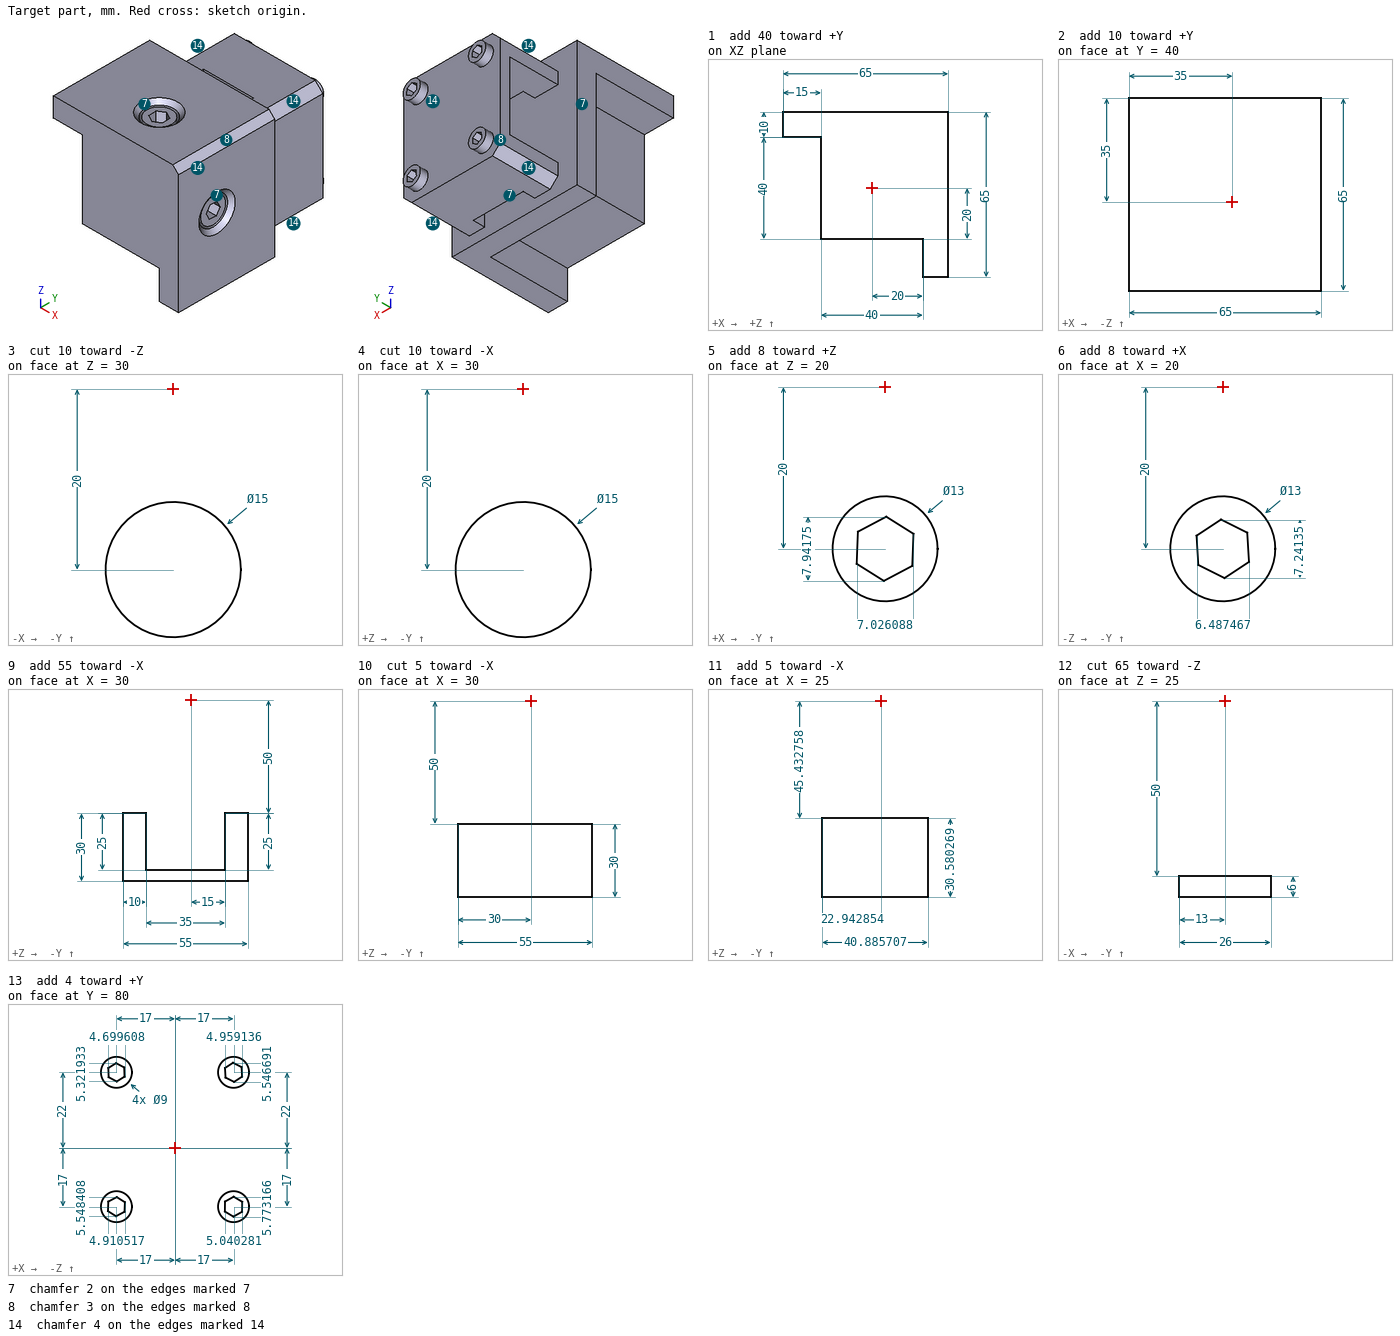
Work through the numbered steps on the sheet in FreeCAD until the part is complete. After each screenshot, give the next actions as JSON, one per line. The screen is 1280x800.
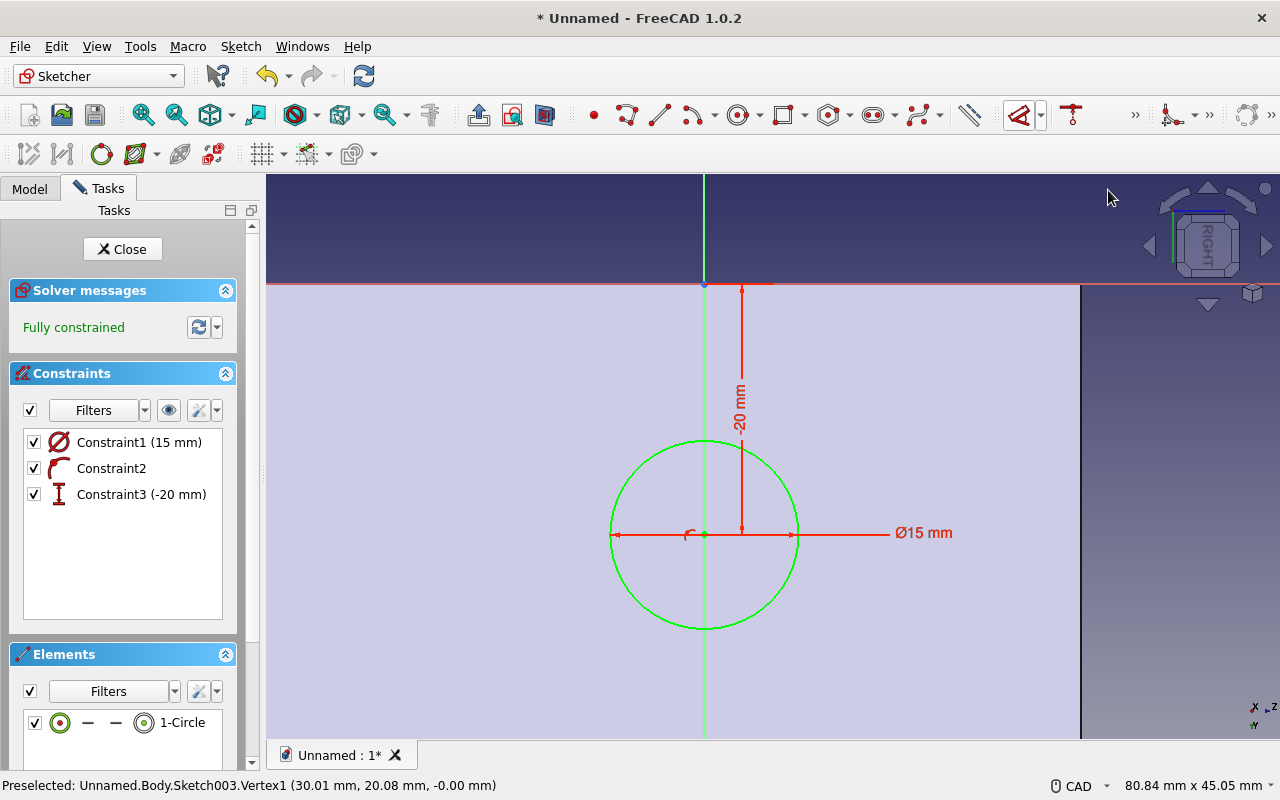
{"action": "left_click", "coordinate": [123, 249]}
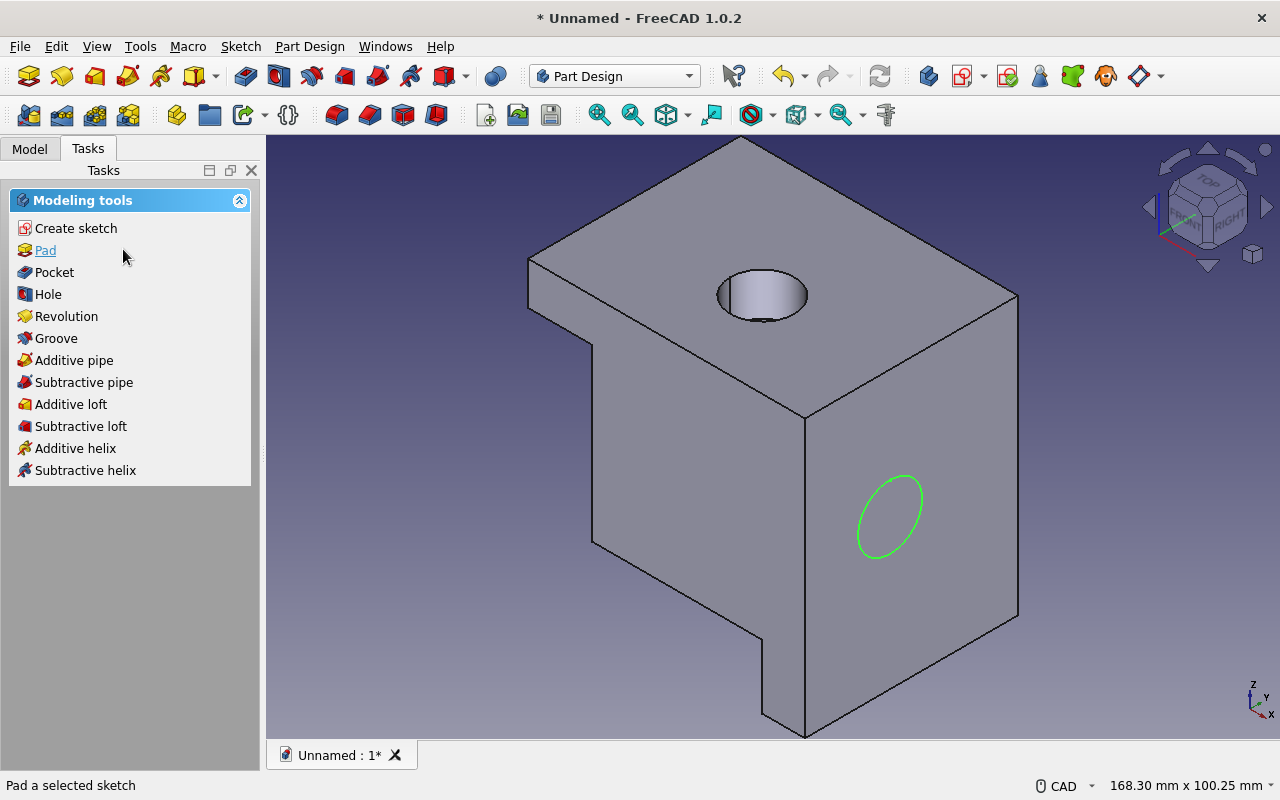
{"action": "left_click", "coordinate": [246, 76]}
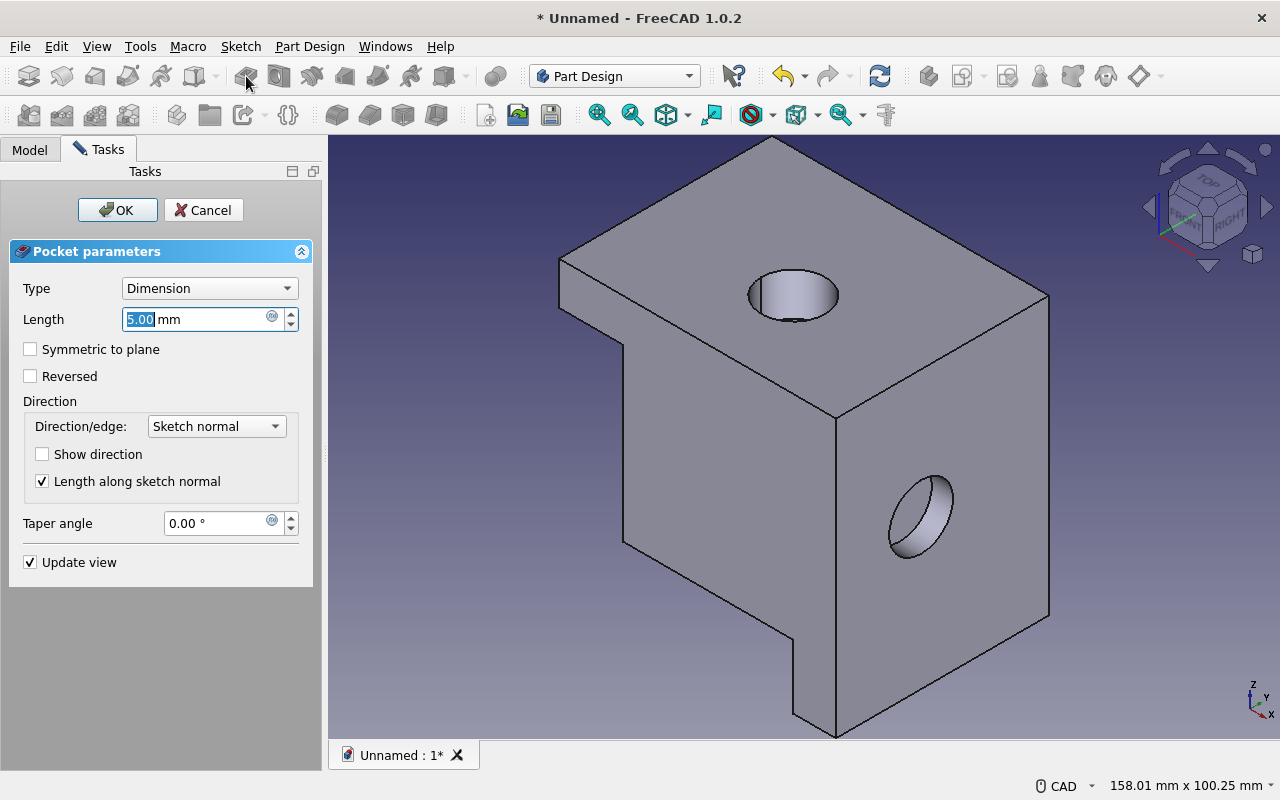
{"action": "type", "text": "10"}
{"action": "key", "text": "Tab"}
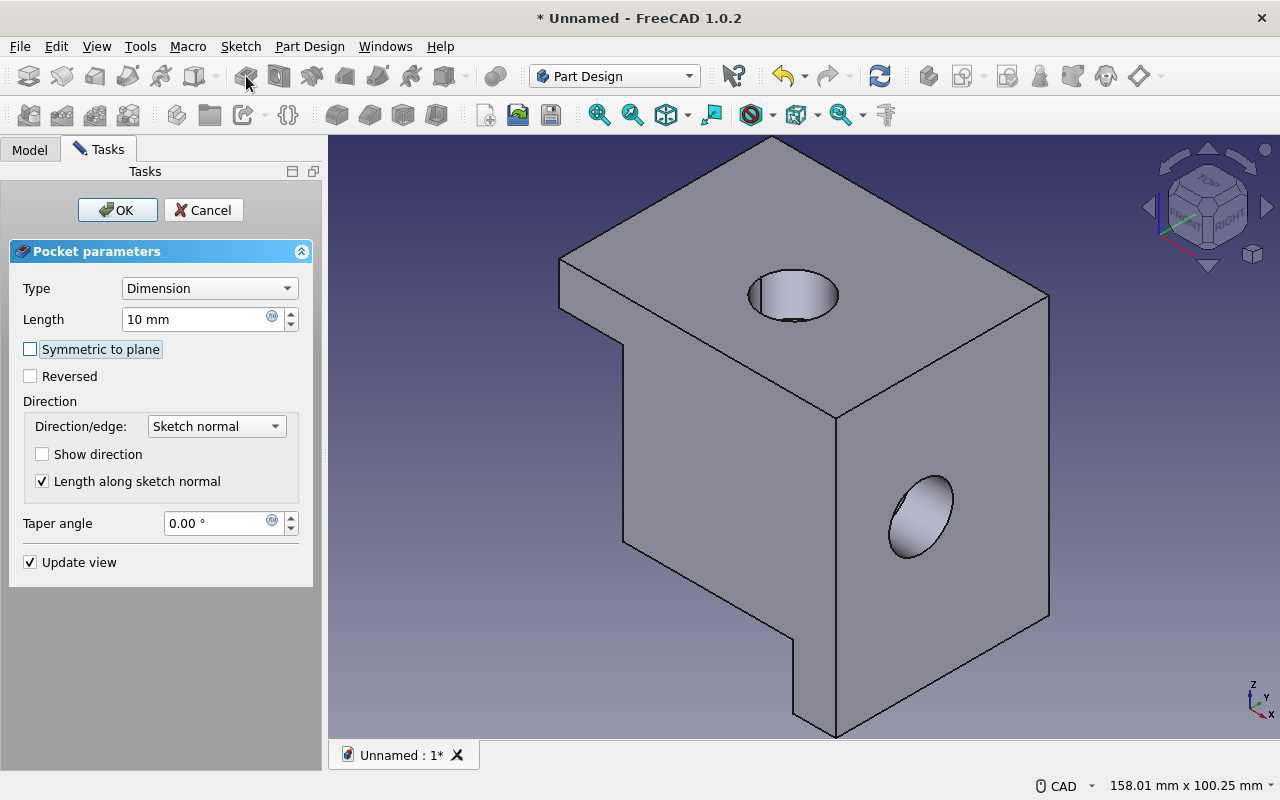
{"action": "left_click", "coordinate": [118, 210]}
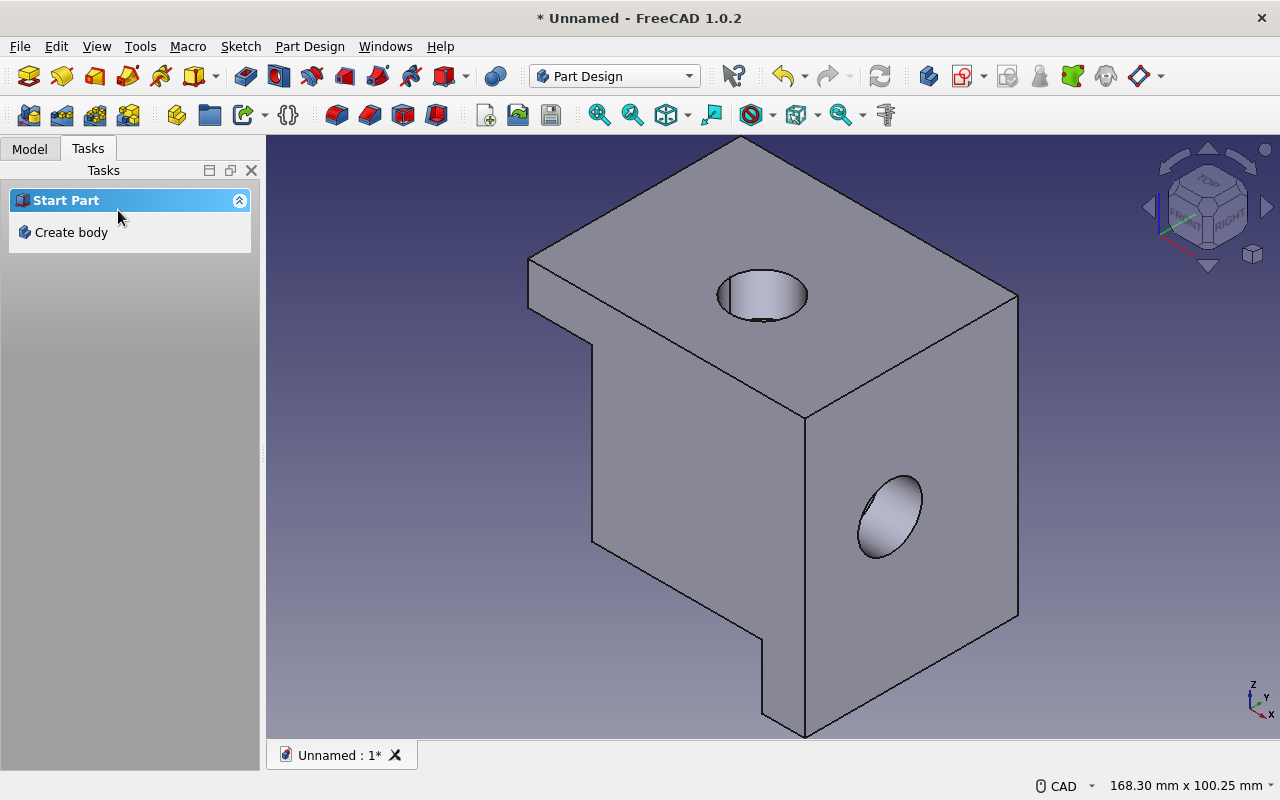
{"action": "key", "text": "5"}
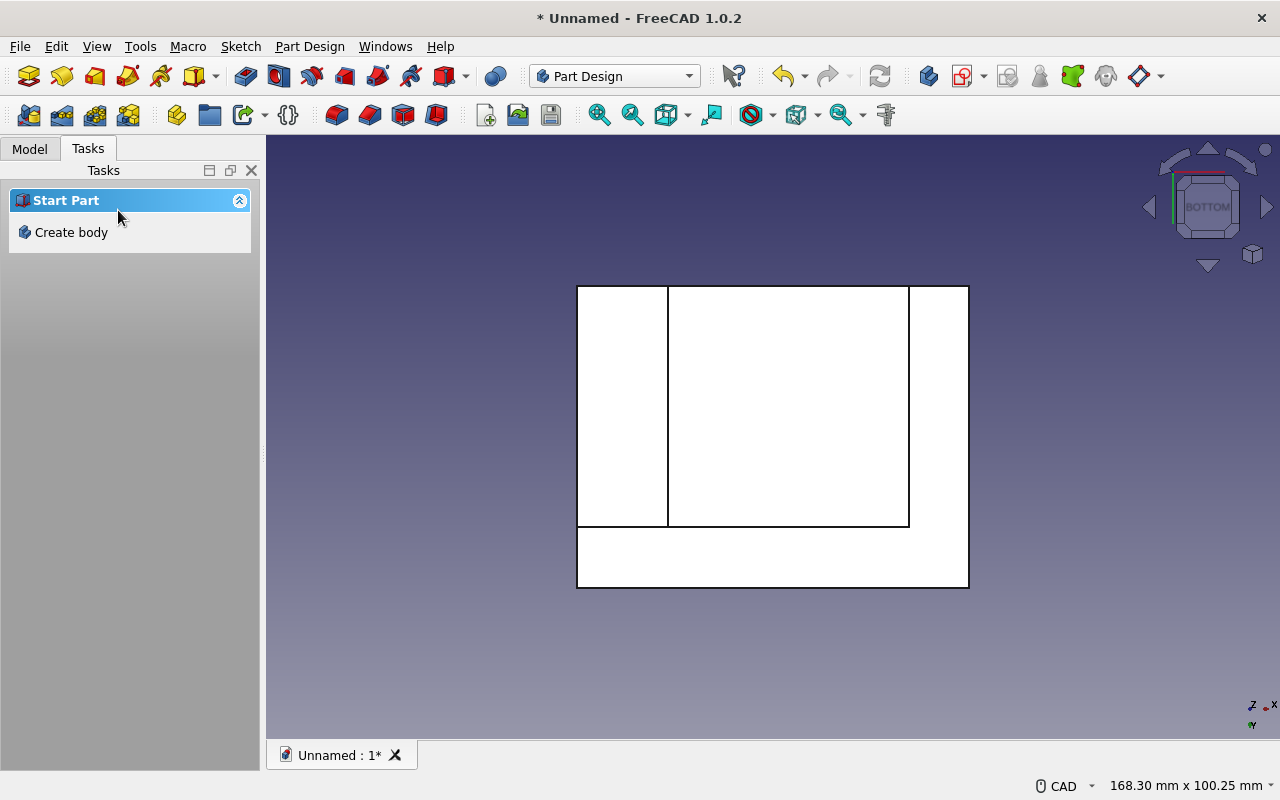
{"action": "left_click", "coordinate": [622, 475]}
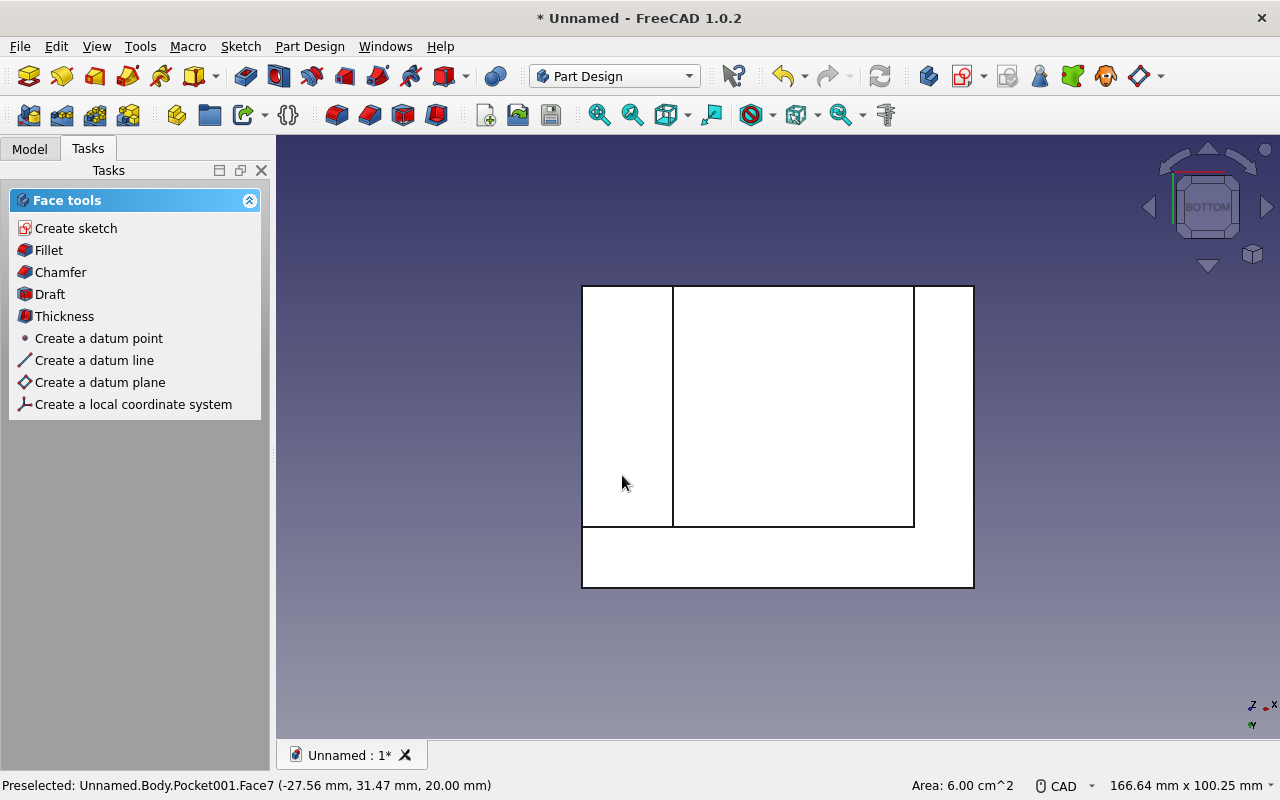
{"action": "left_click", "coordinate": [962, 76]}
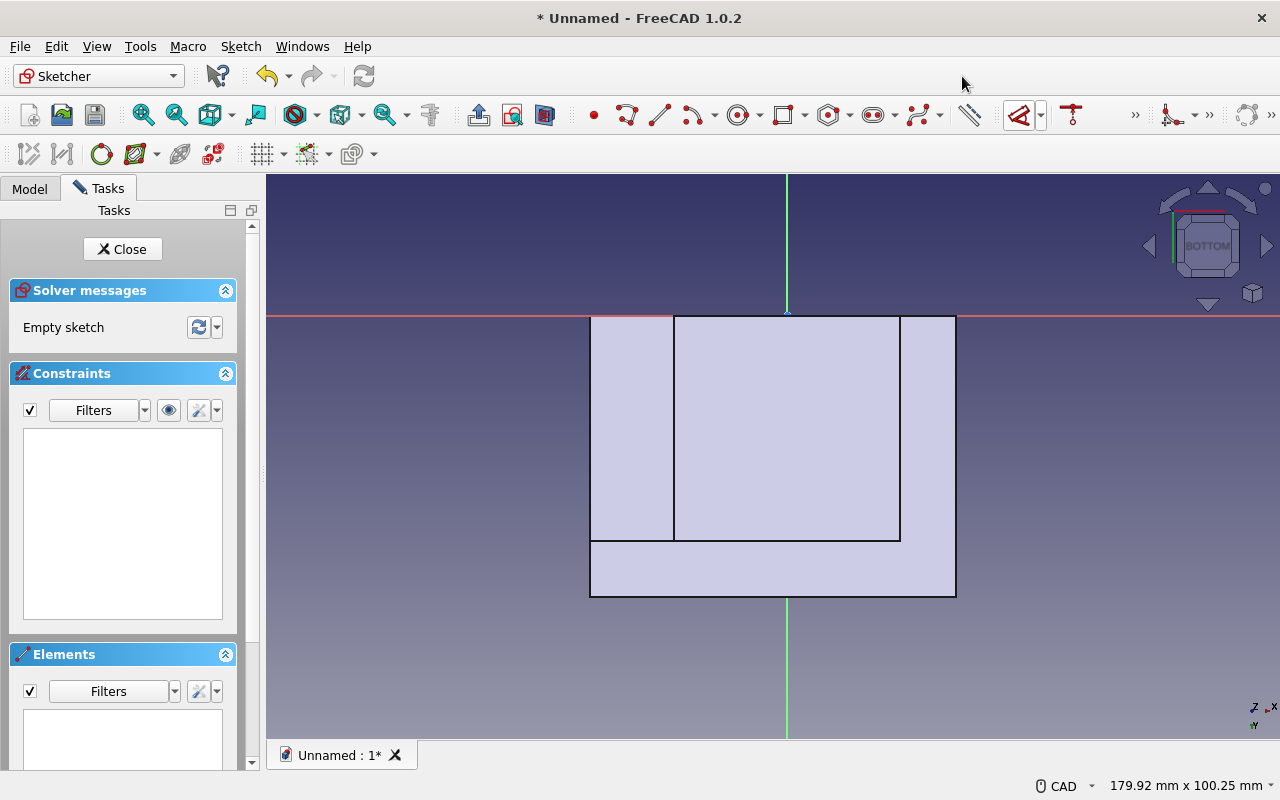
{"action": "scroll", "coordinate": [854, 336], "scroll_direction": "up", "scroll_amount": 4}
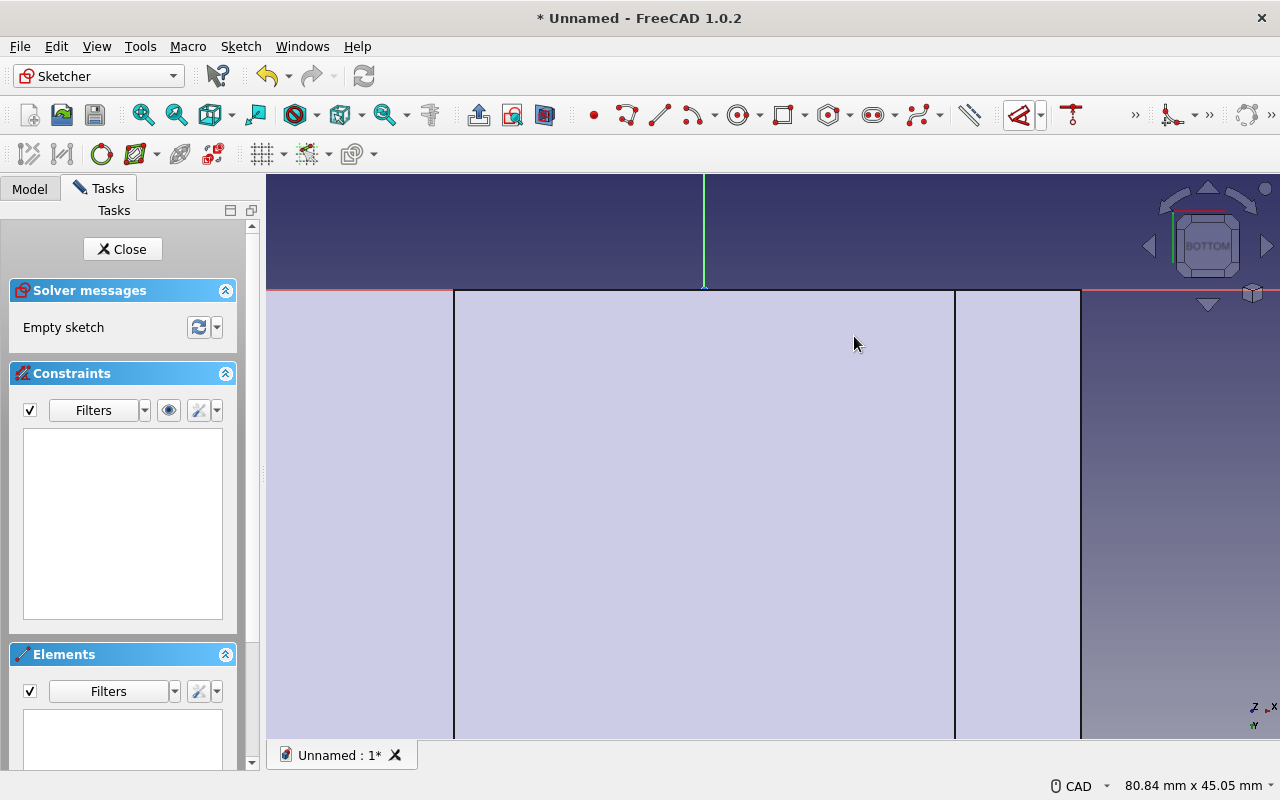
{"action": "left_click", "coordinate": [828, 116]}